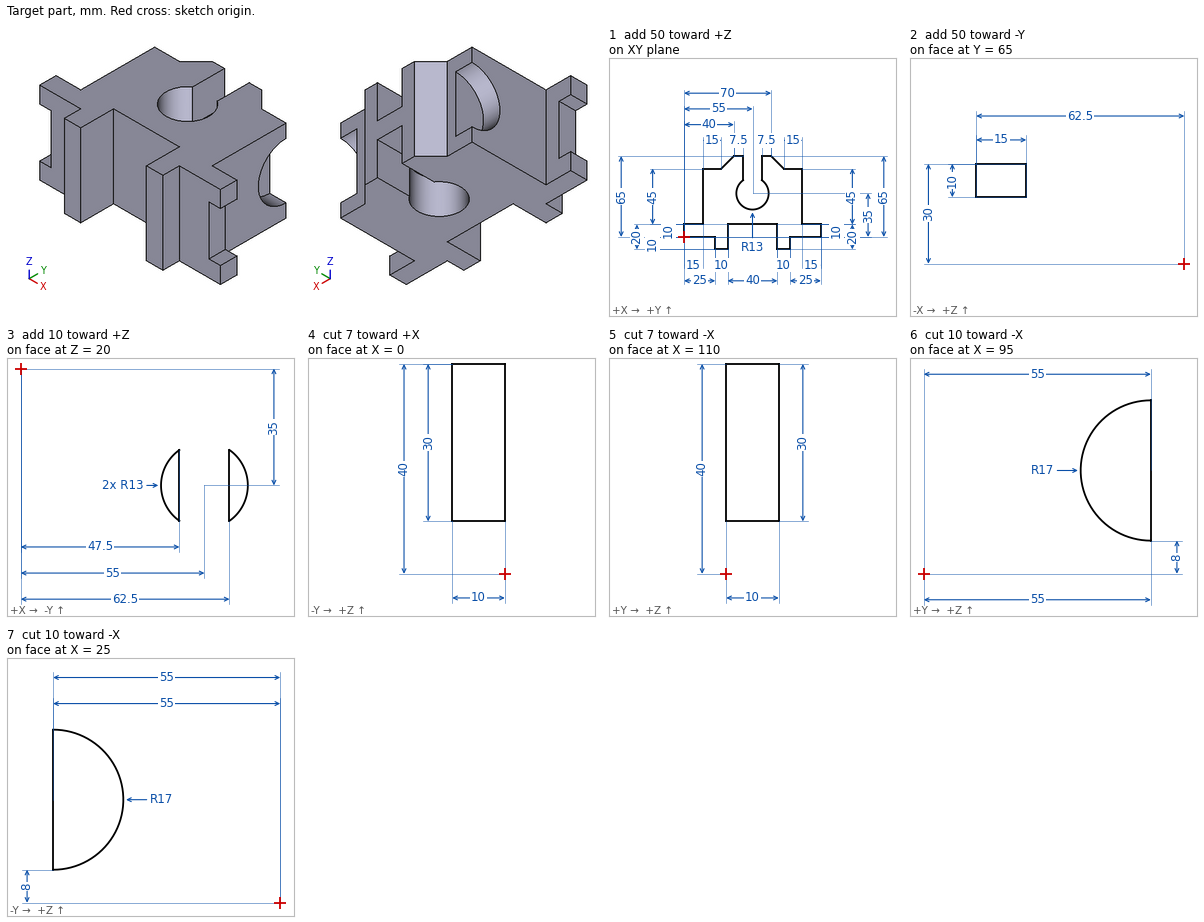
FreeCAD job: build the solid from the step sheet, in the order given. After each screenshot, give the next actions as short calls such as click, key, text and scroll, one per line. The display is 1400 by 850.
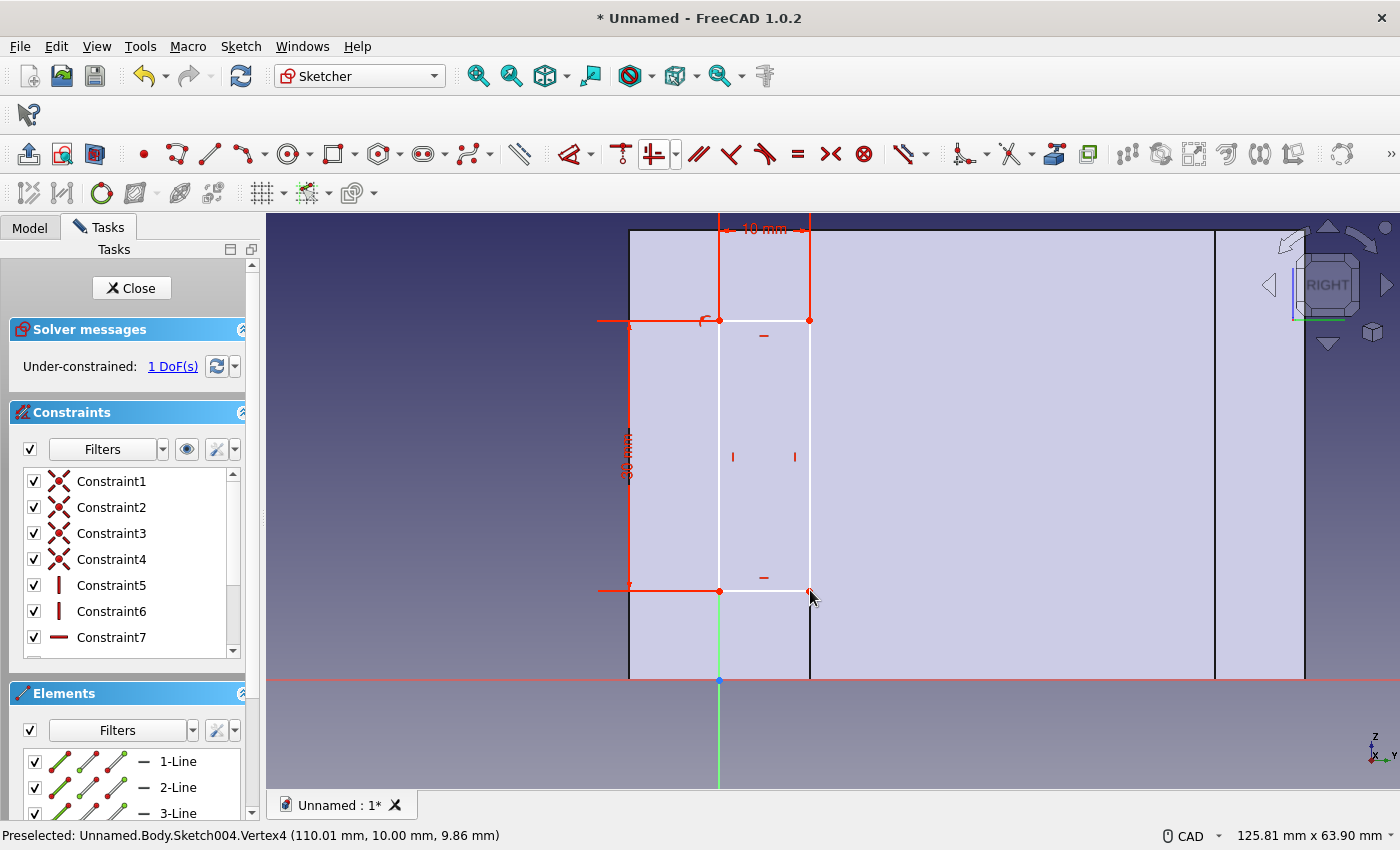
click(568, 154)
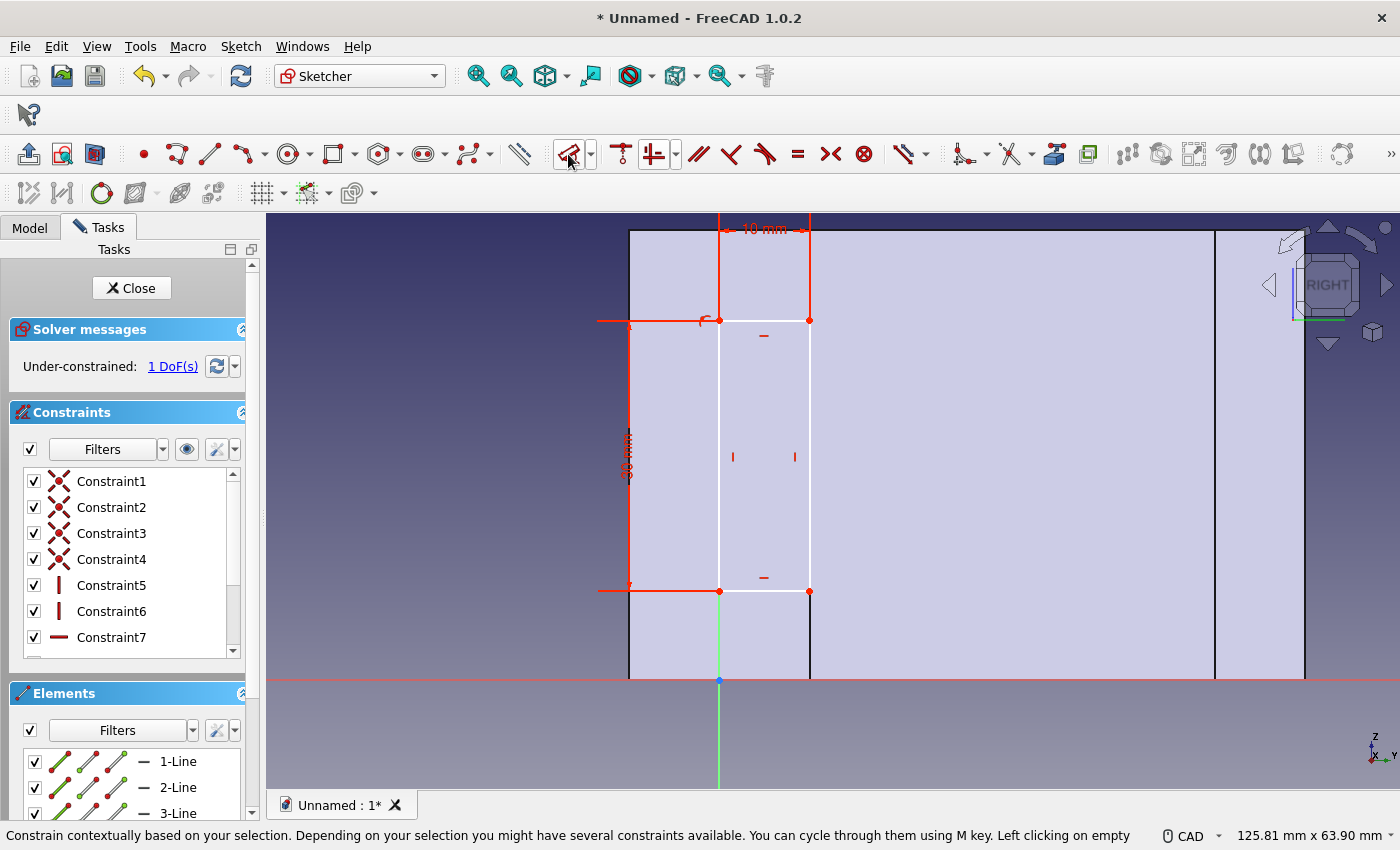
click(719, 321)
click(685, 501)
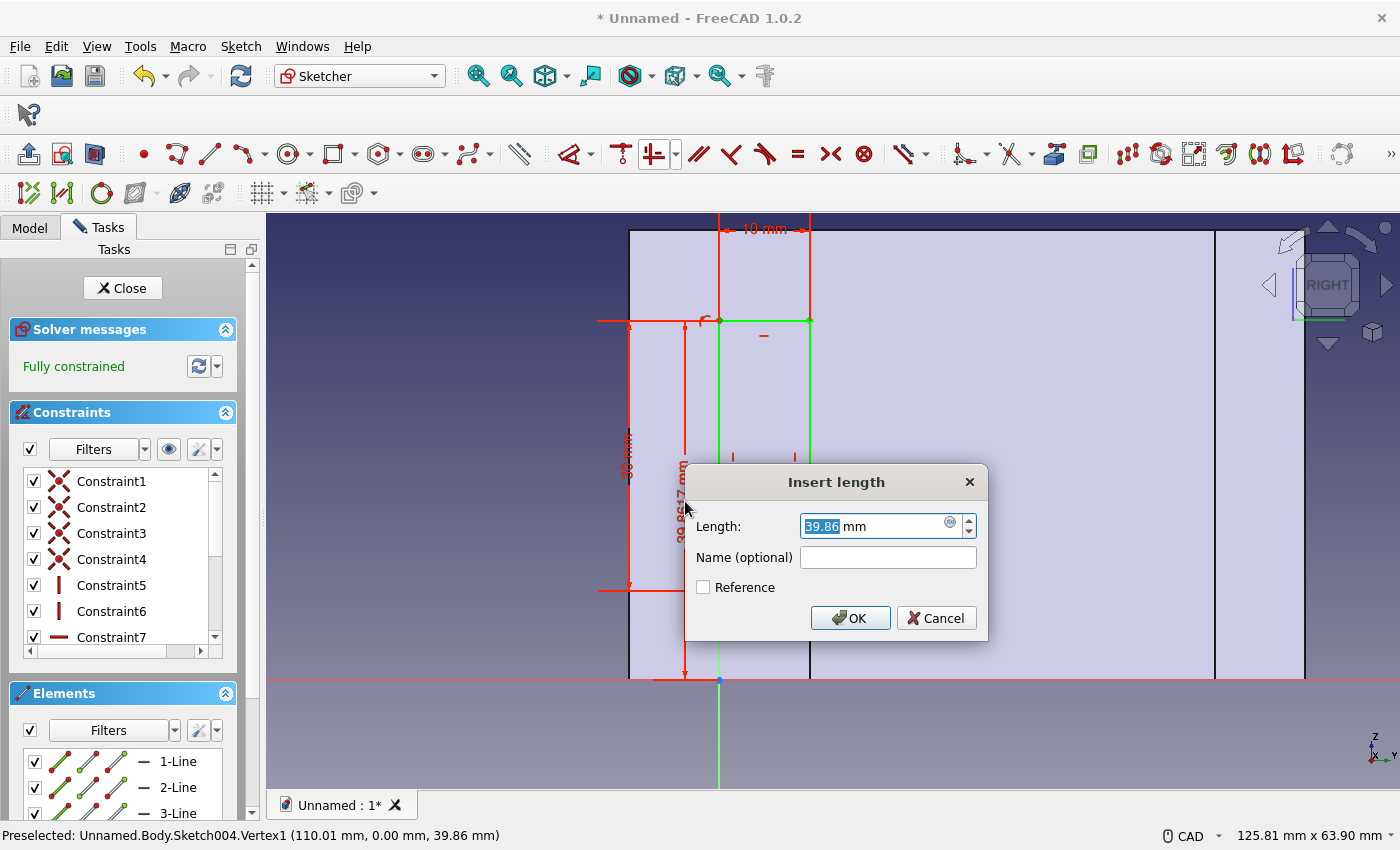
text(40)
key(Return)
key(Escape)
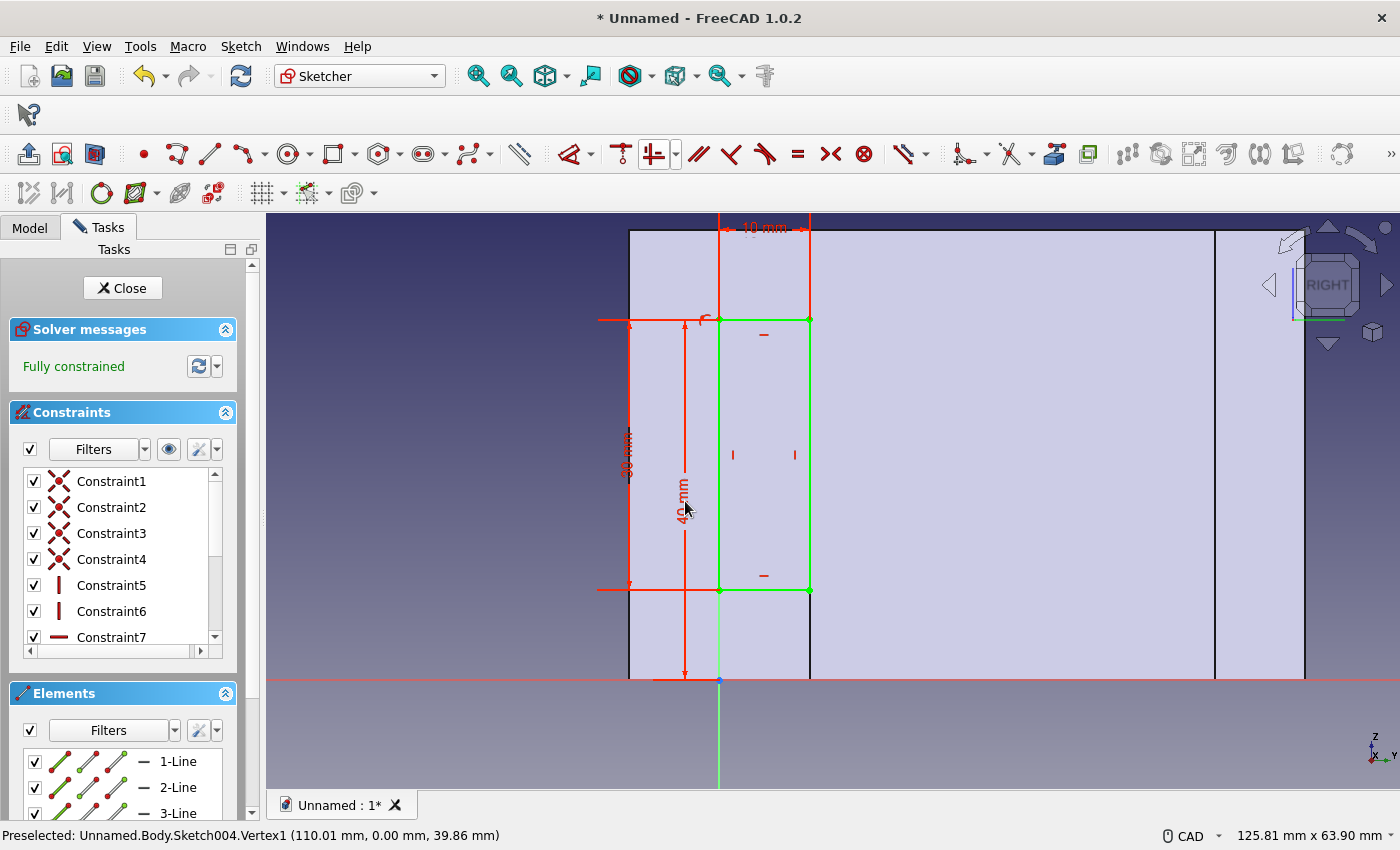
click(123, 288)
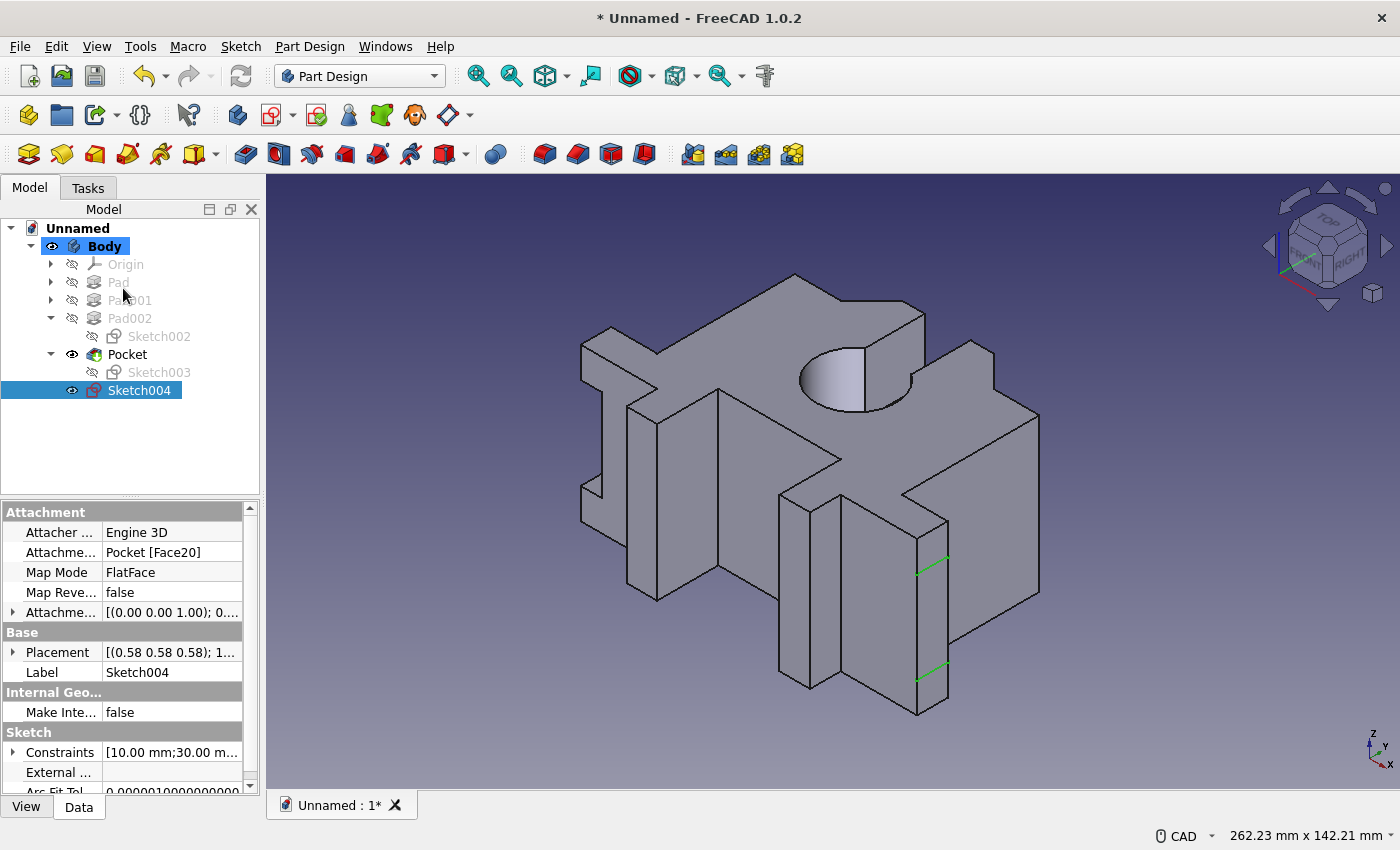
click(246, 154)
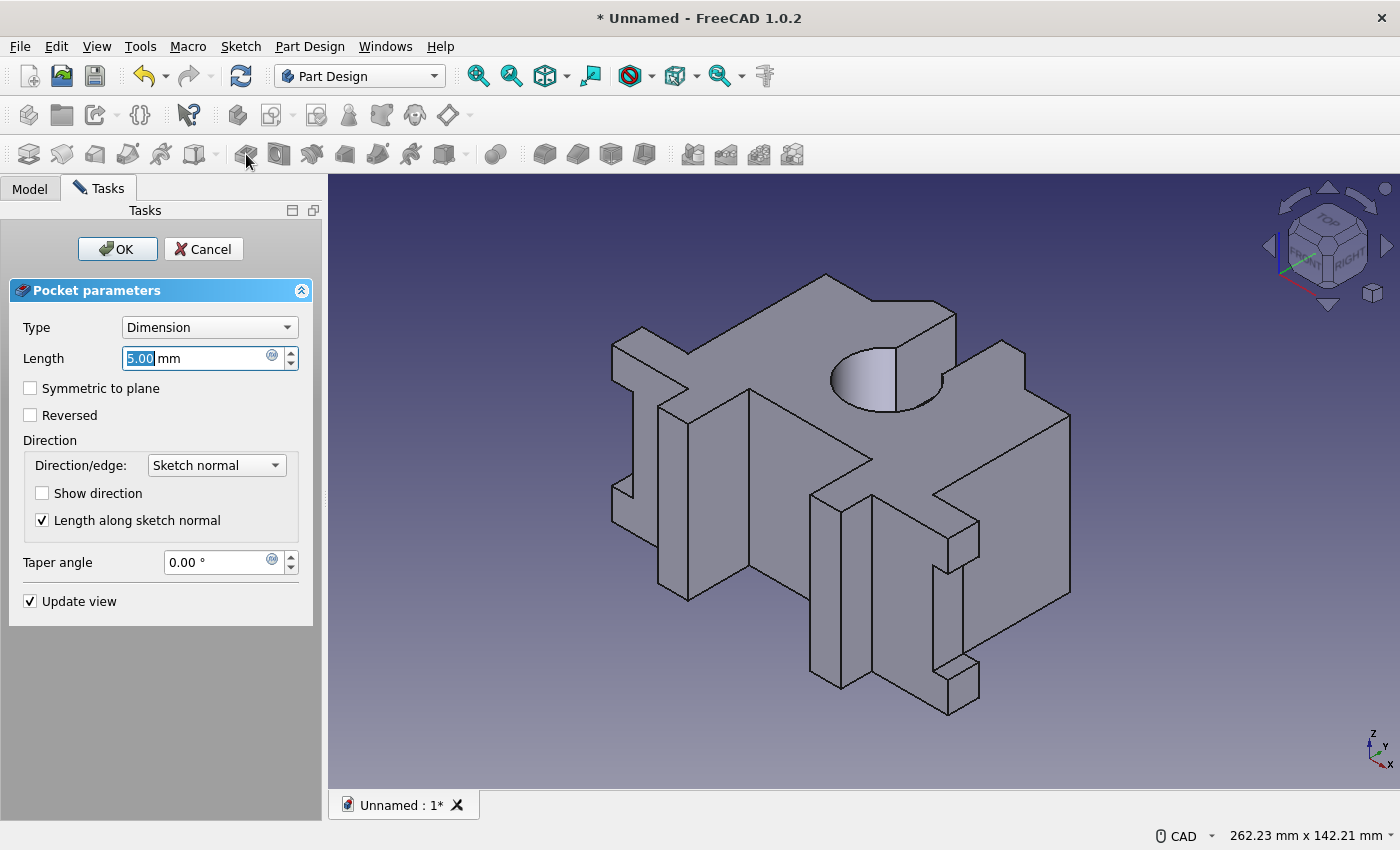
text(7)
key(Tab)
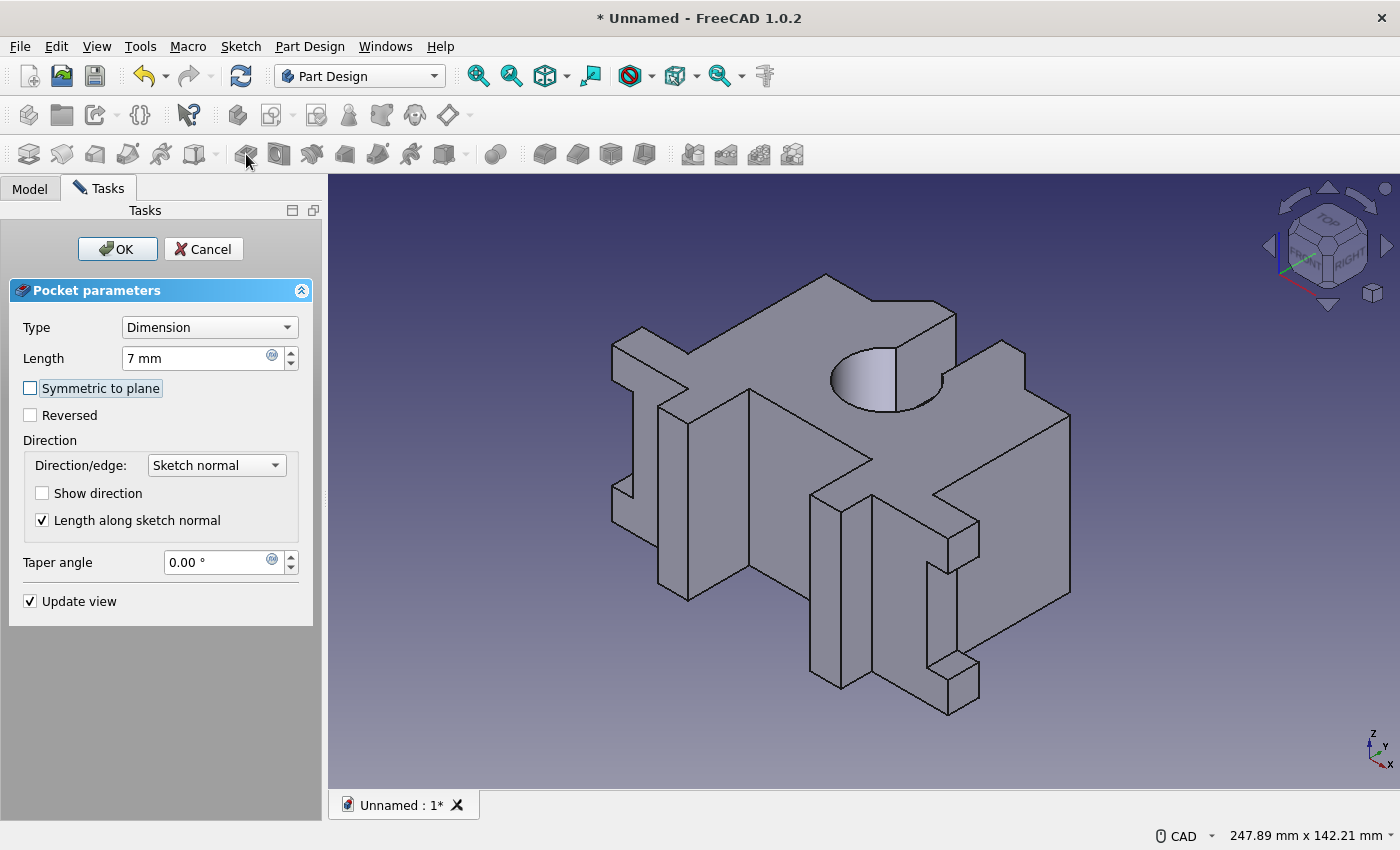
click(118, 249)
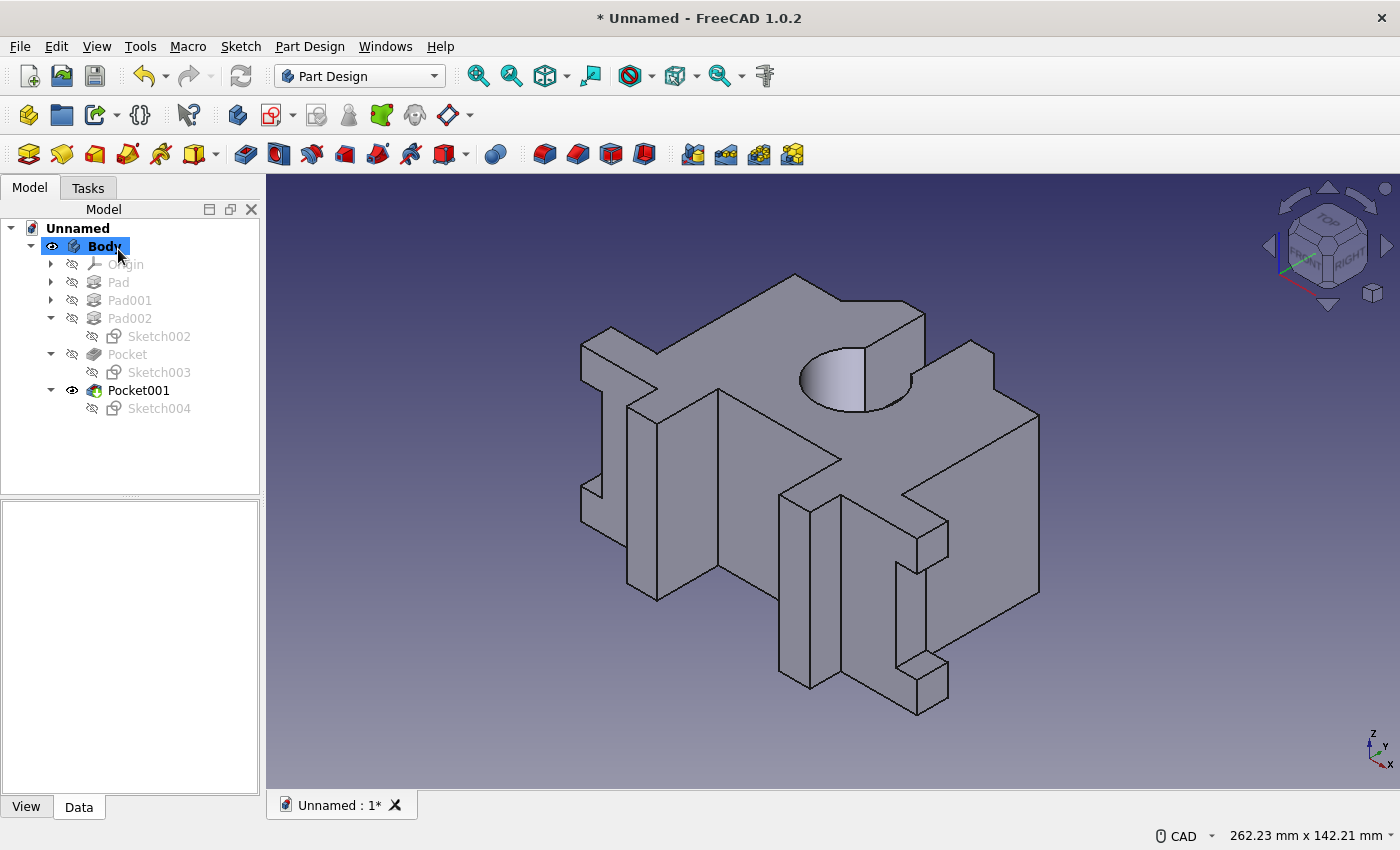
click(971, 542)